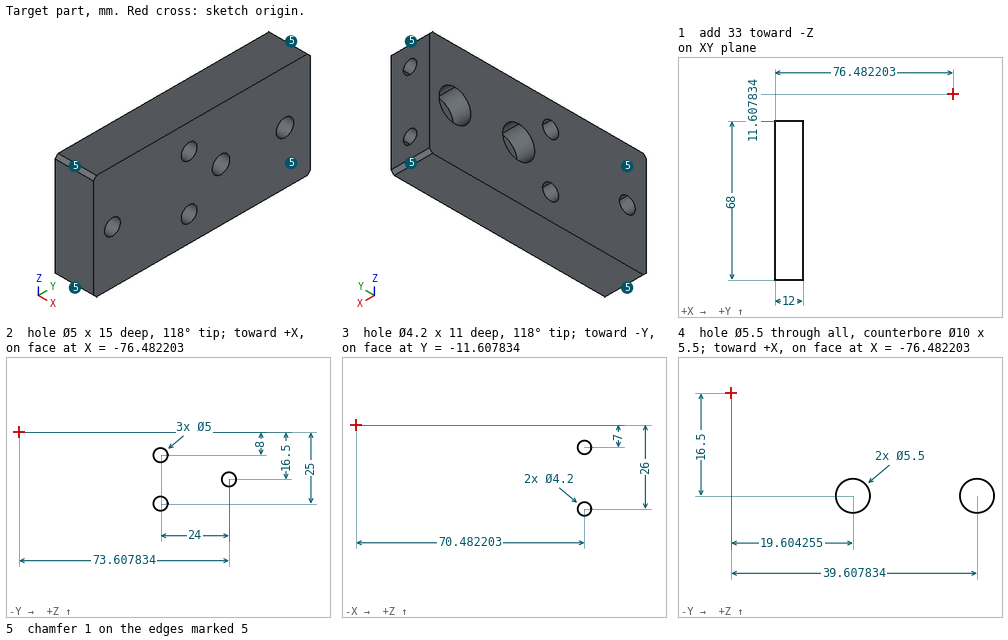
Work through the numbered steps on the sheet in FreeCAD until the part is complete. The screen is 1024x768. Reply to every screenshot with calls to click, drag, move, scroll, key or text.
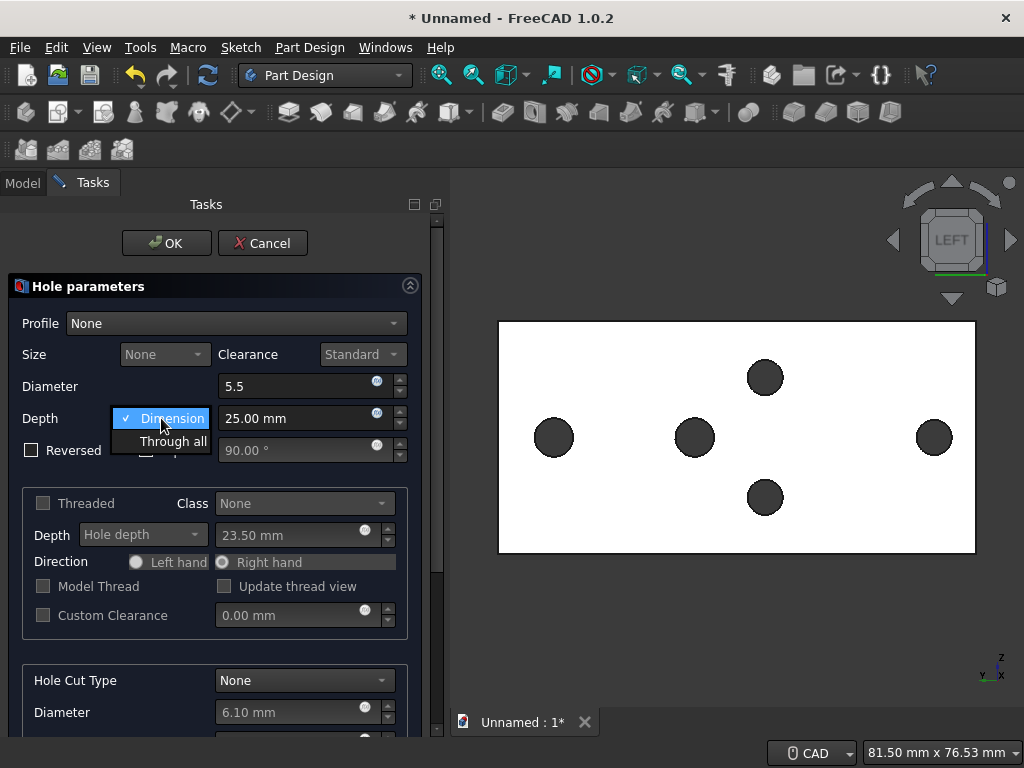
click(160, 442)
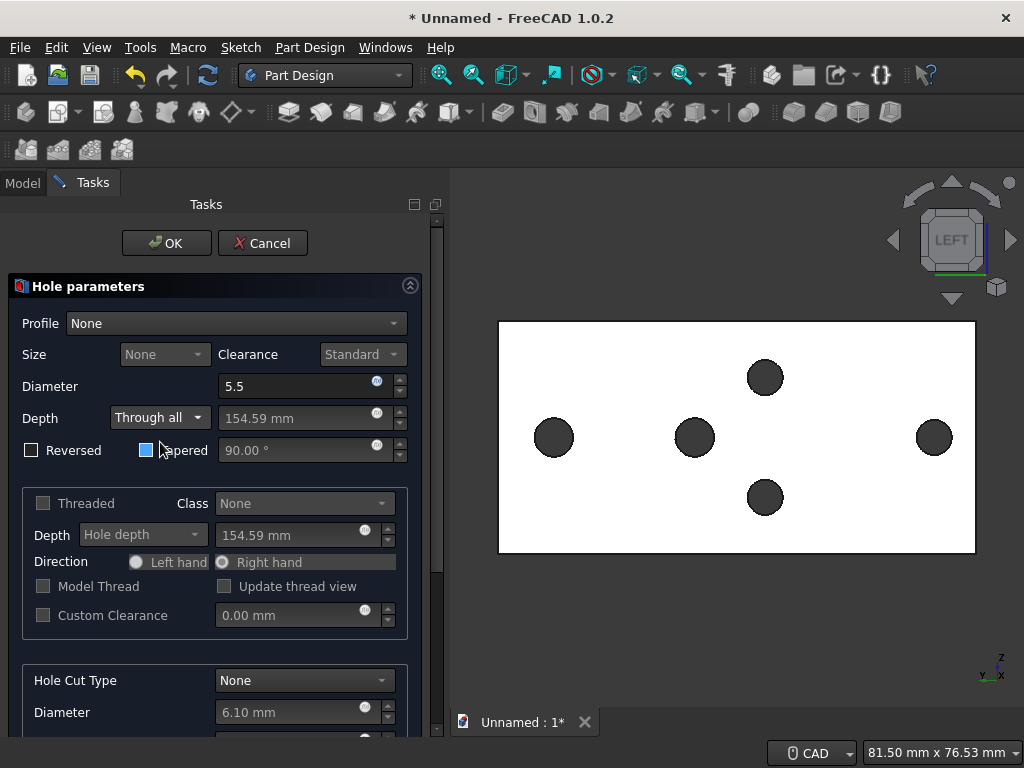
click(306, 680)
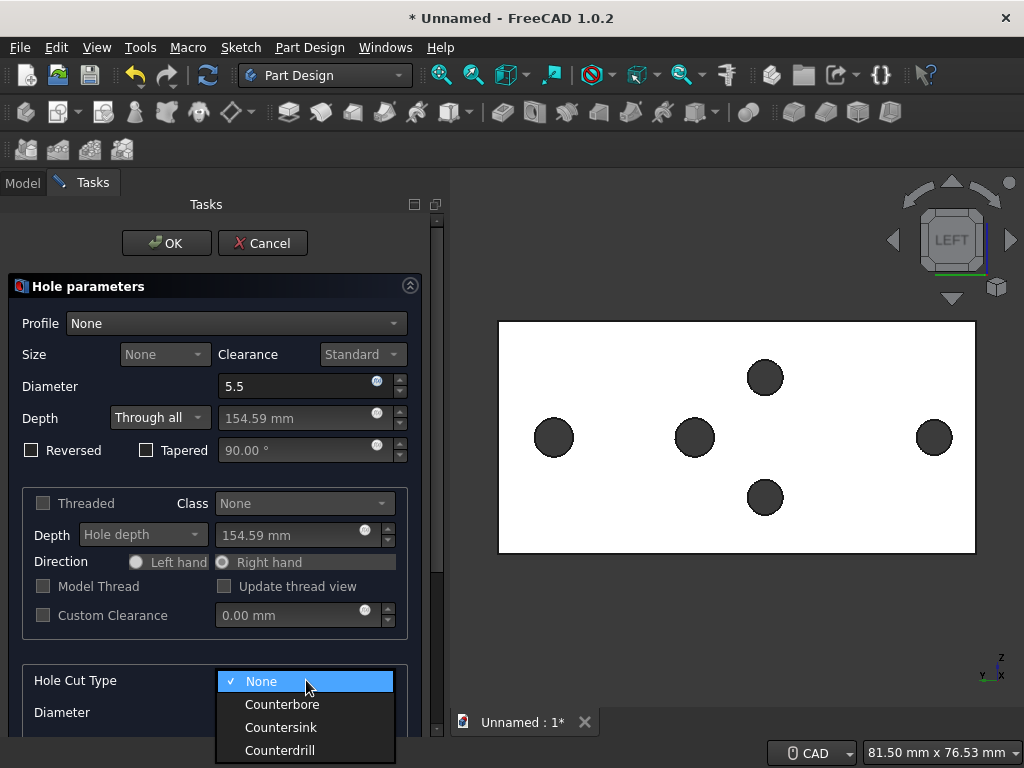
click(304, 704)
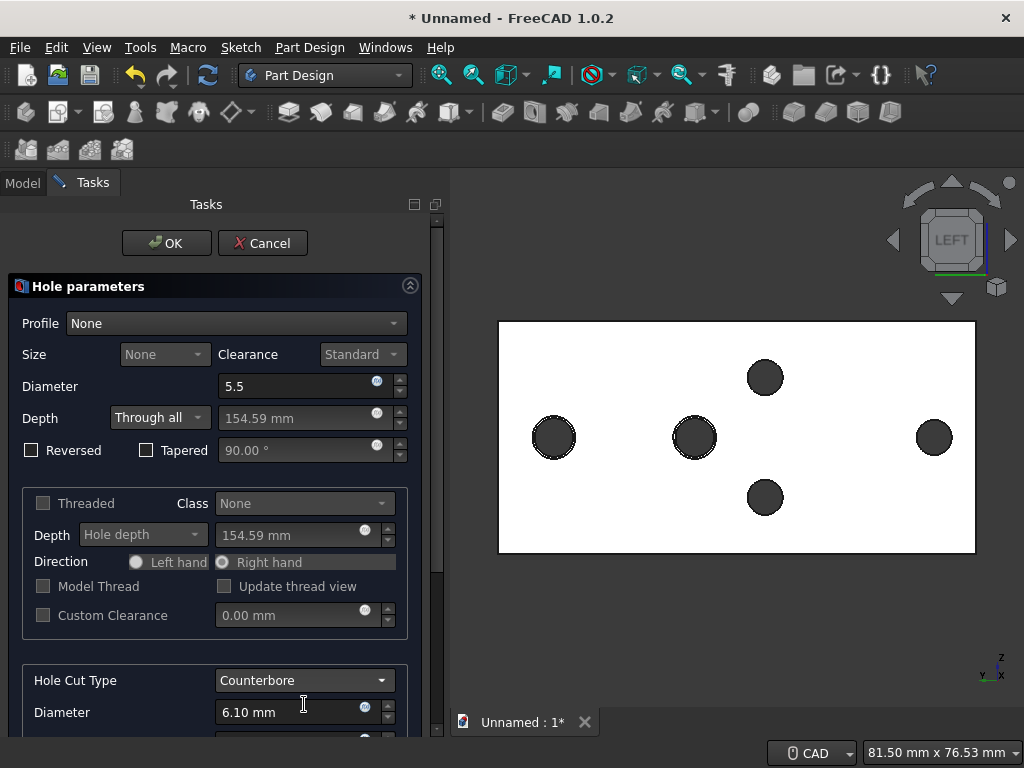
triple_click(298, 712)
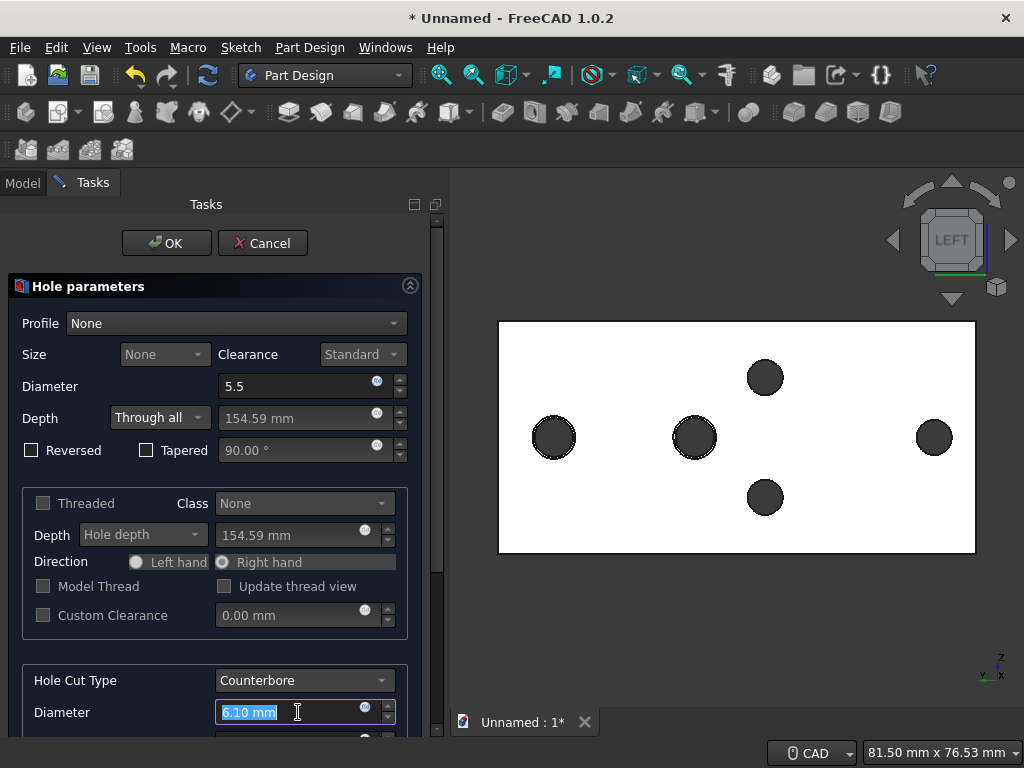
text(10)
key(Tab)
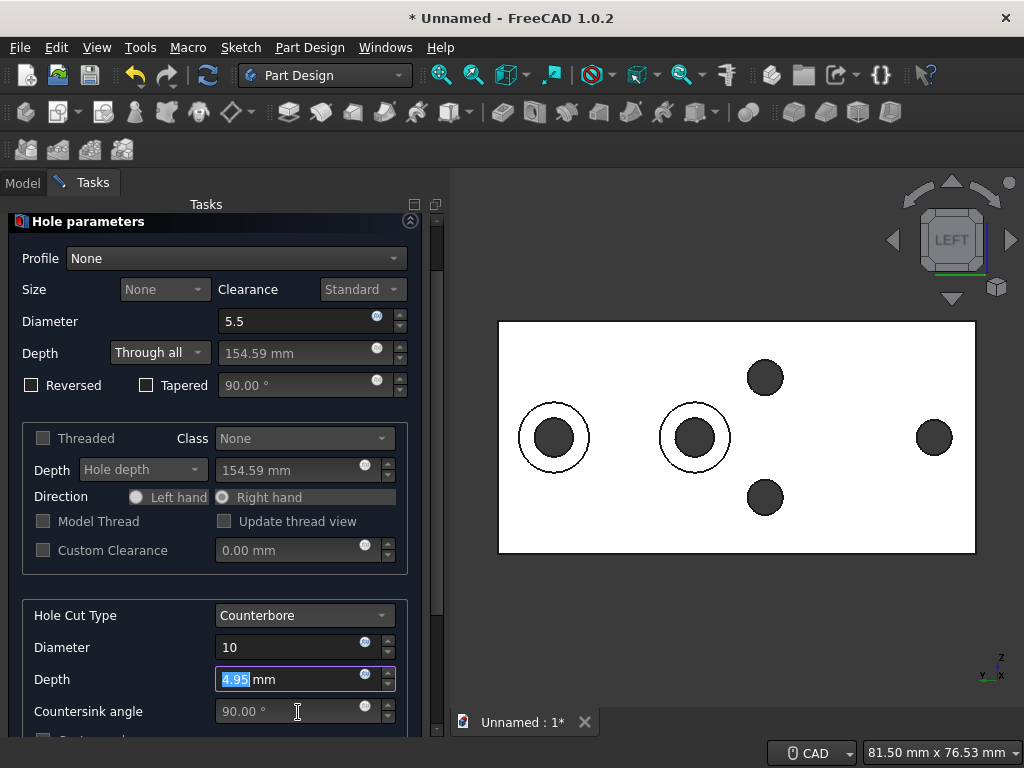
text(5.5)
key(Tab)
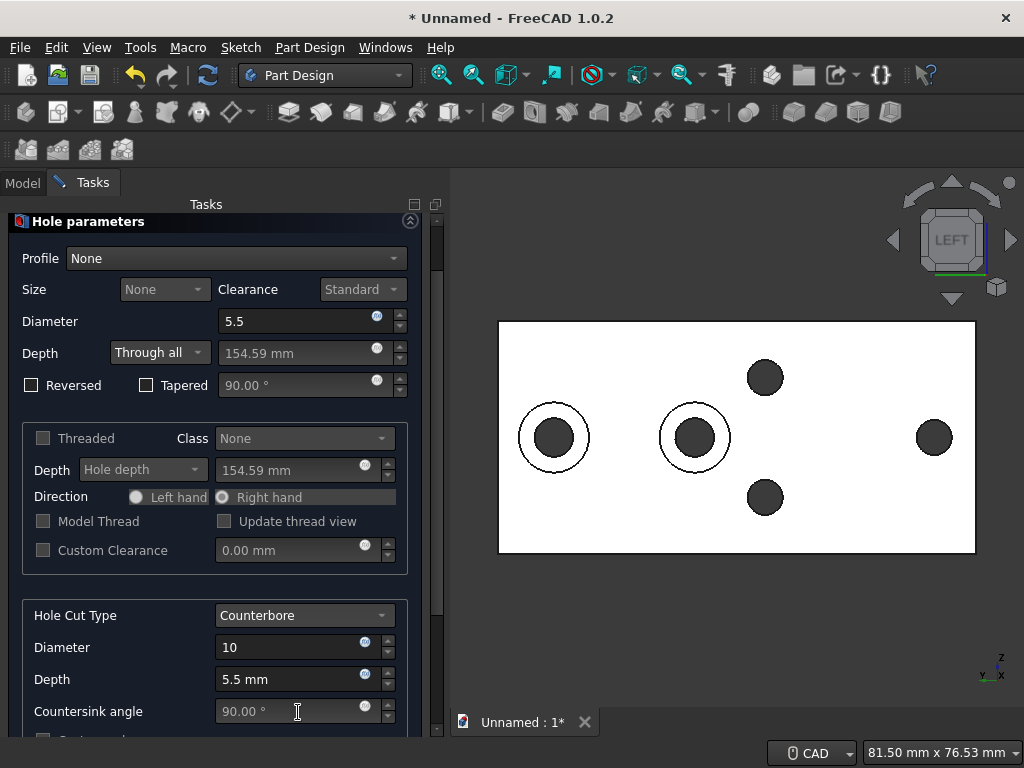
scroll(437, 475, up, 2)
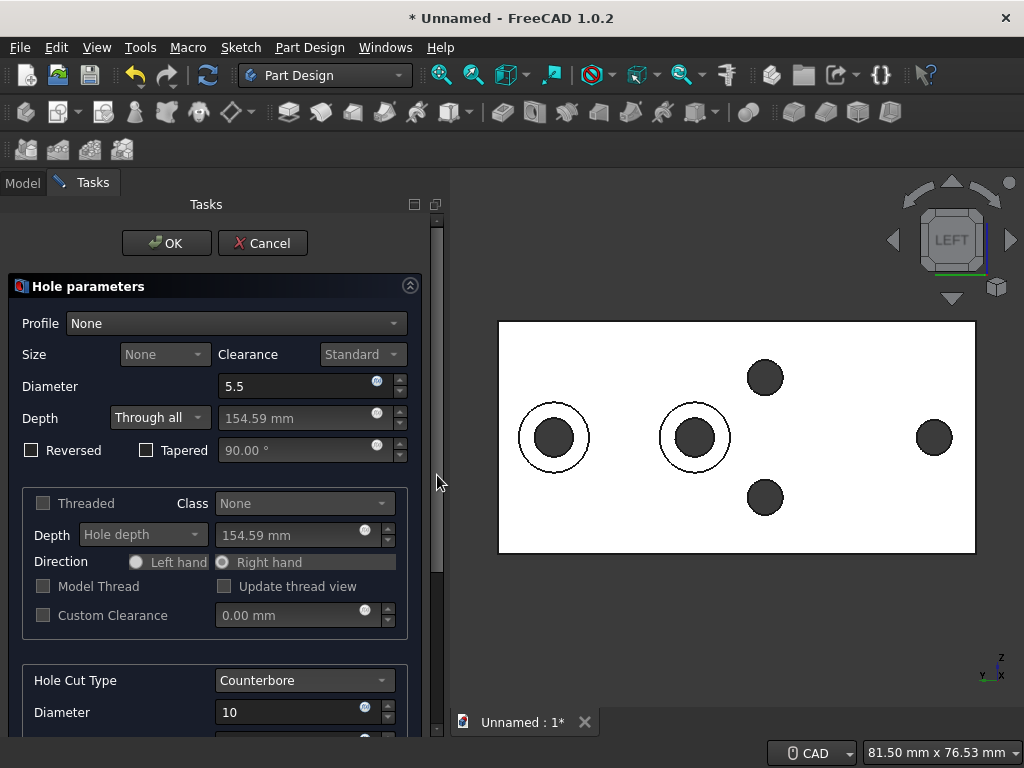
click(167, 243)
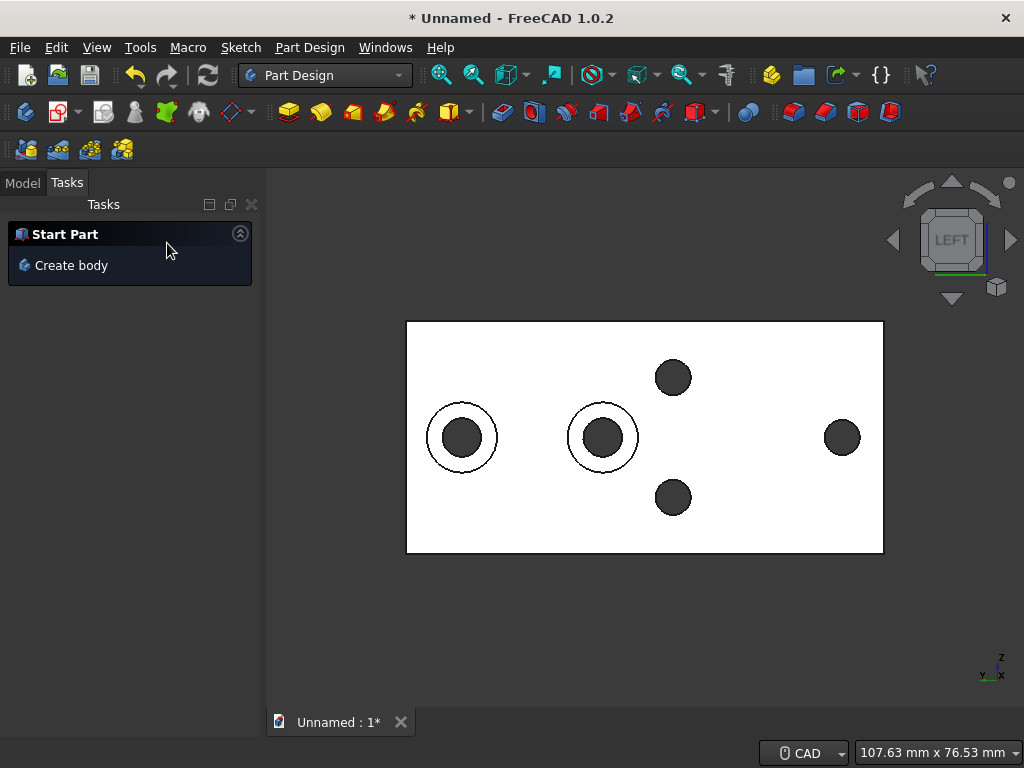
key(0)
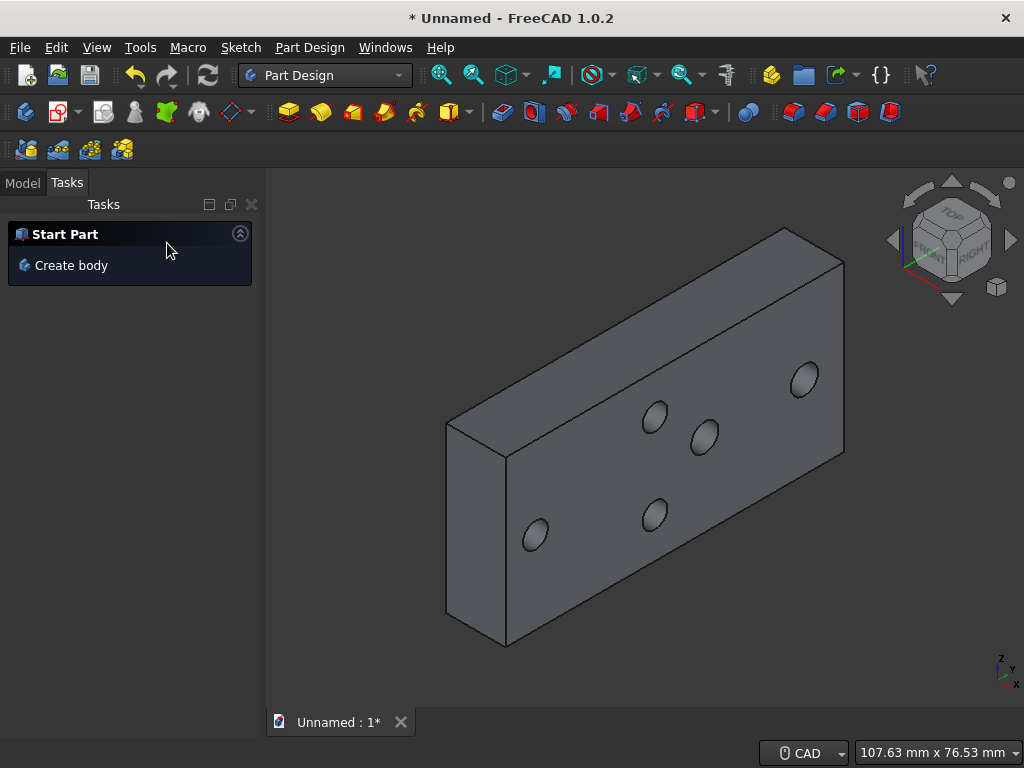
click(476, 439)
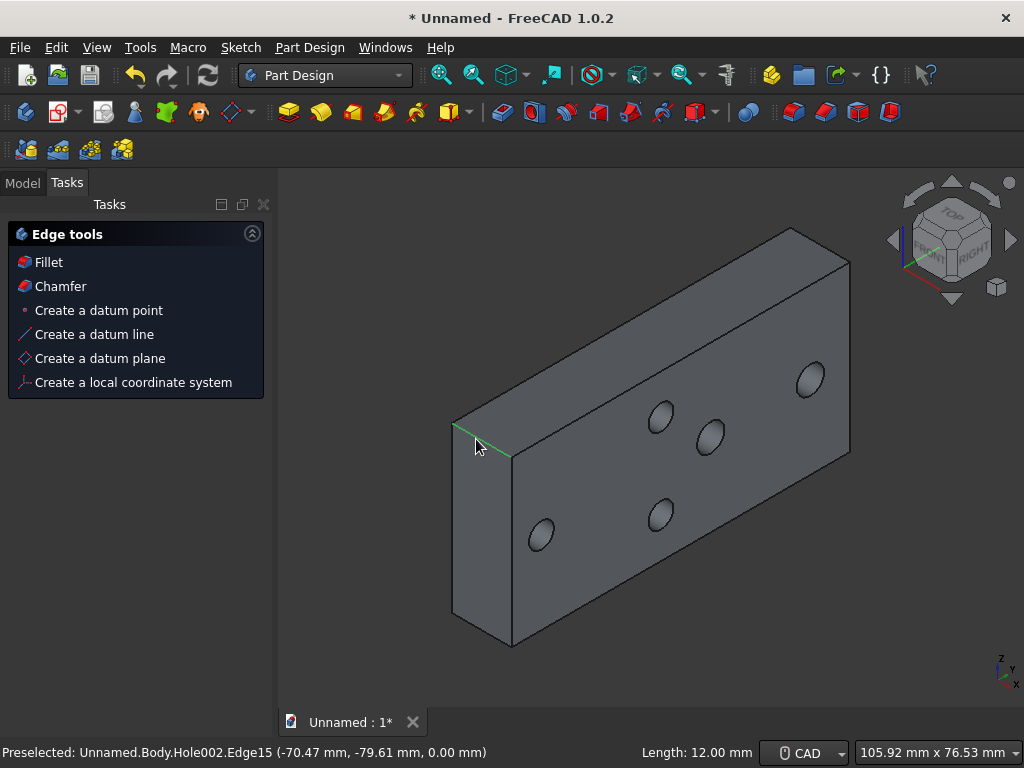
key(2)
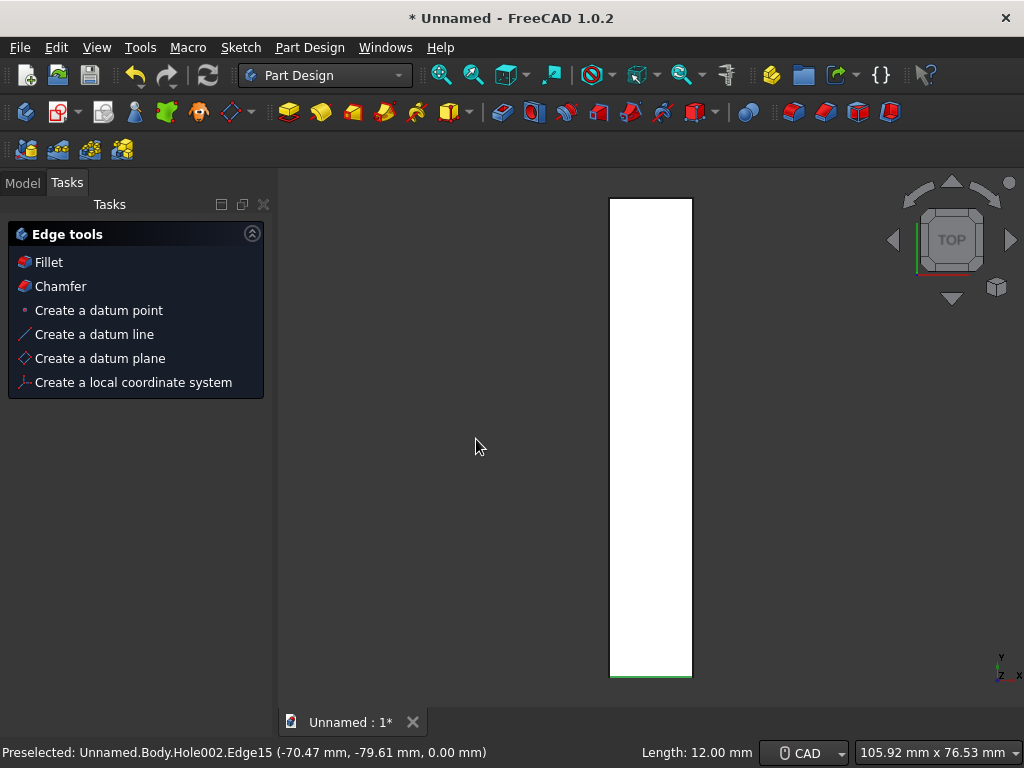
click(651, 197, ctrl)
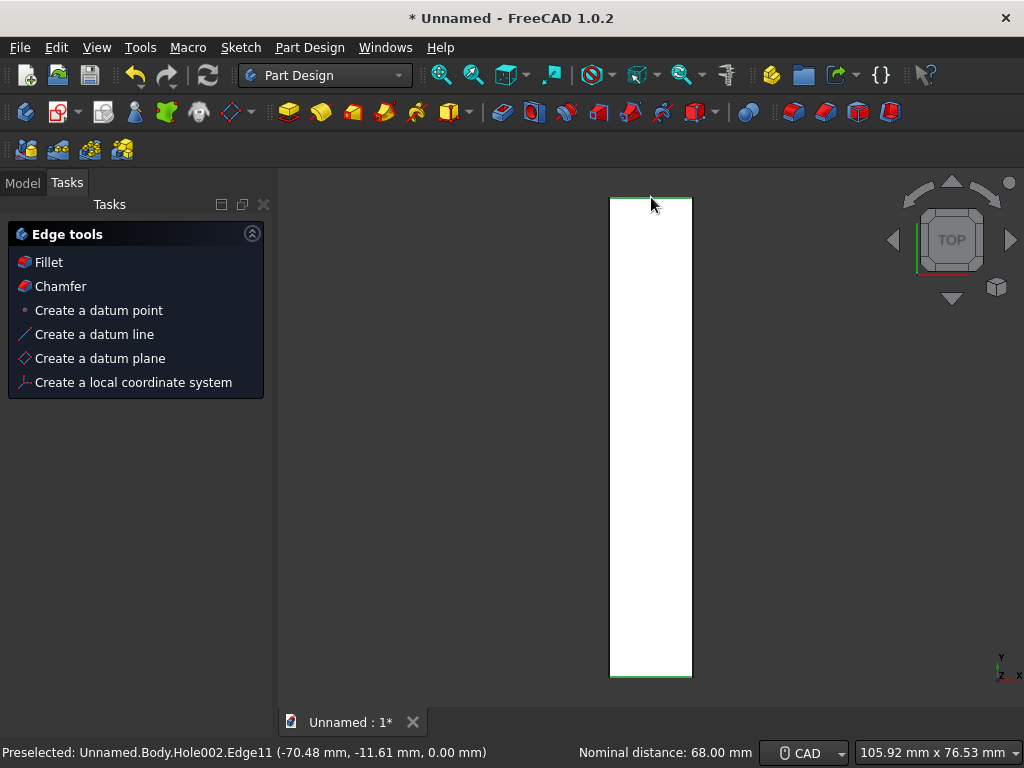
key(1)